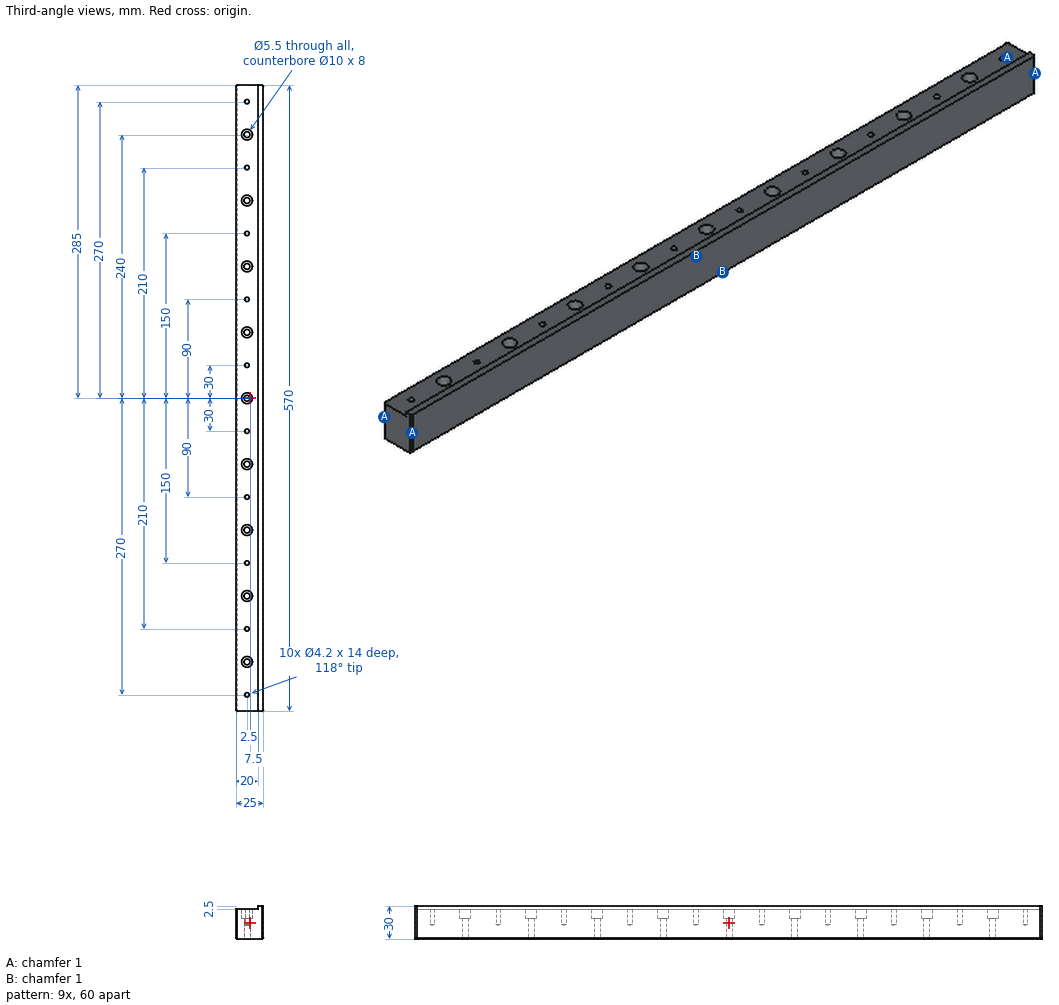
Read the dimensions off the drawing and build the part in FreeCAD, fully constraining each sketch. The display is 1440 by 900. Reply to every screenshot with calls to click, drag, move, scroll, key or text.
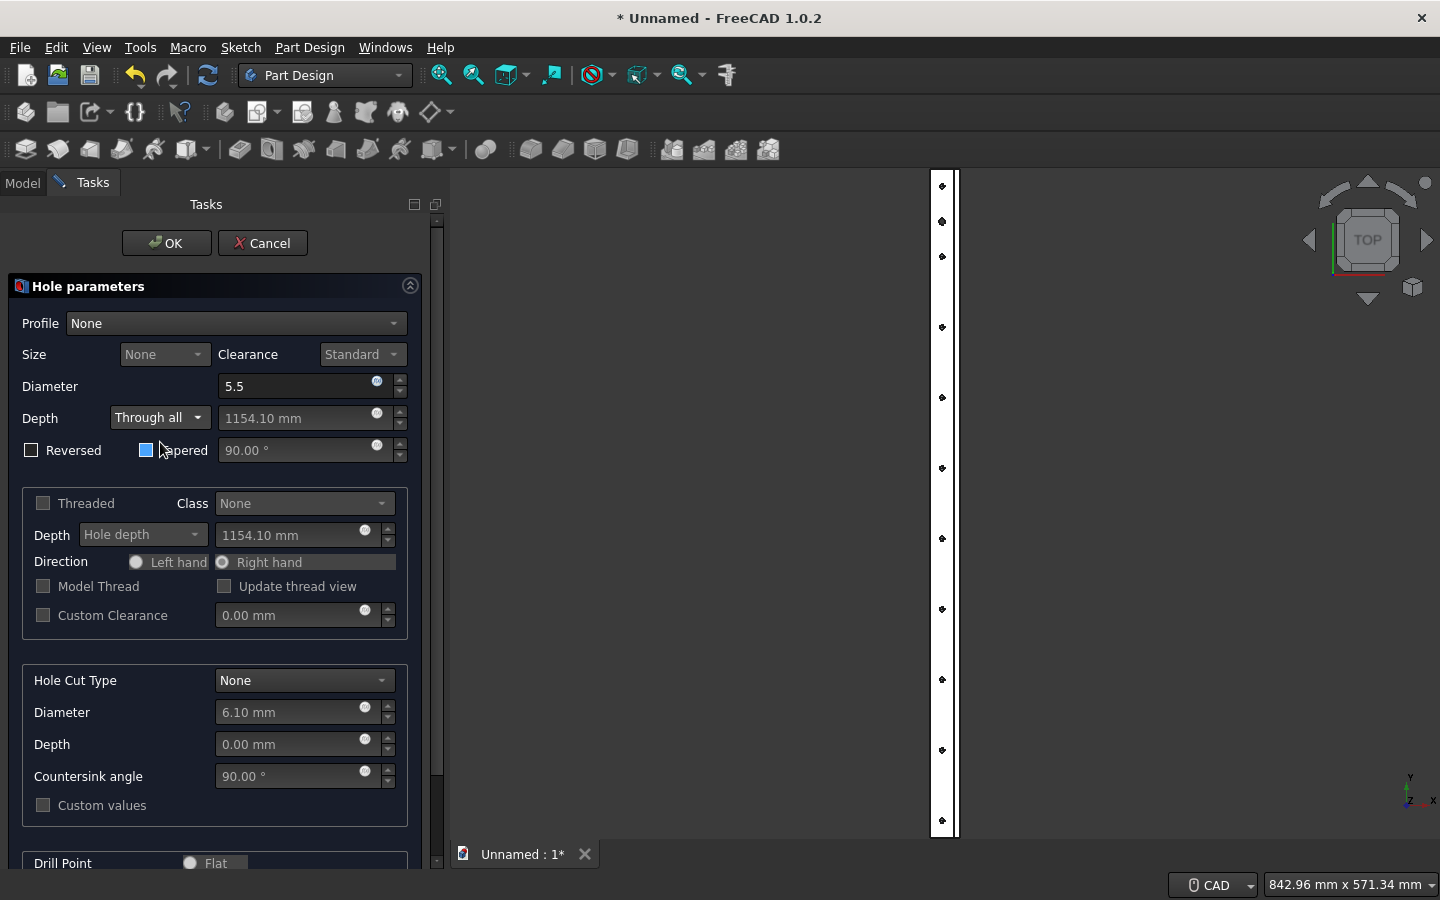
click(306, 680)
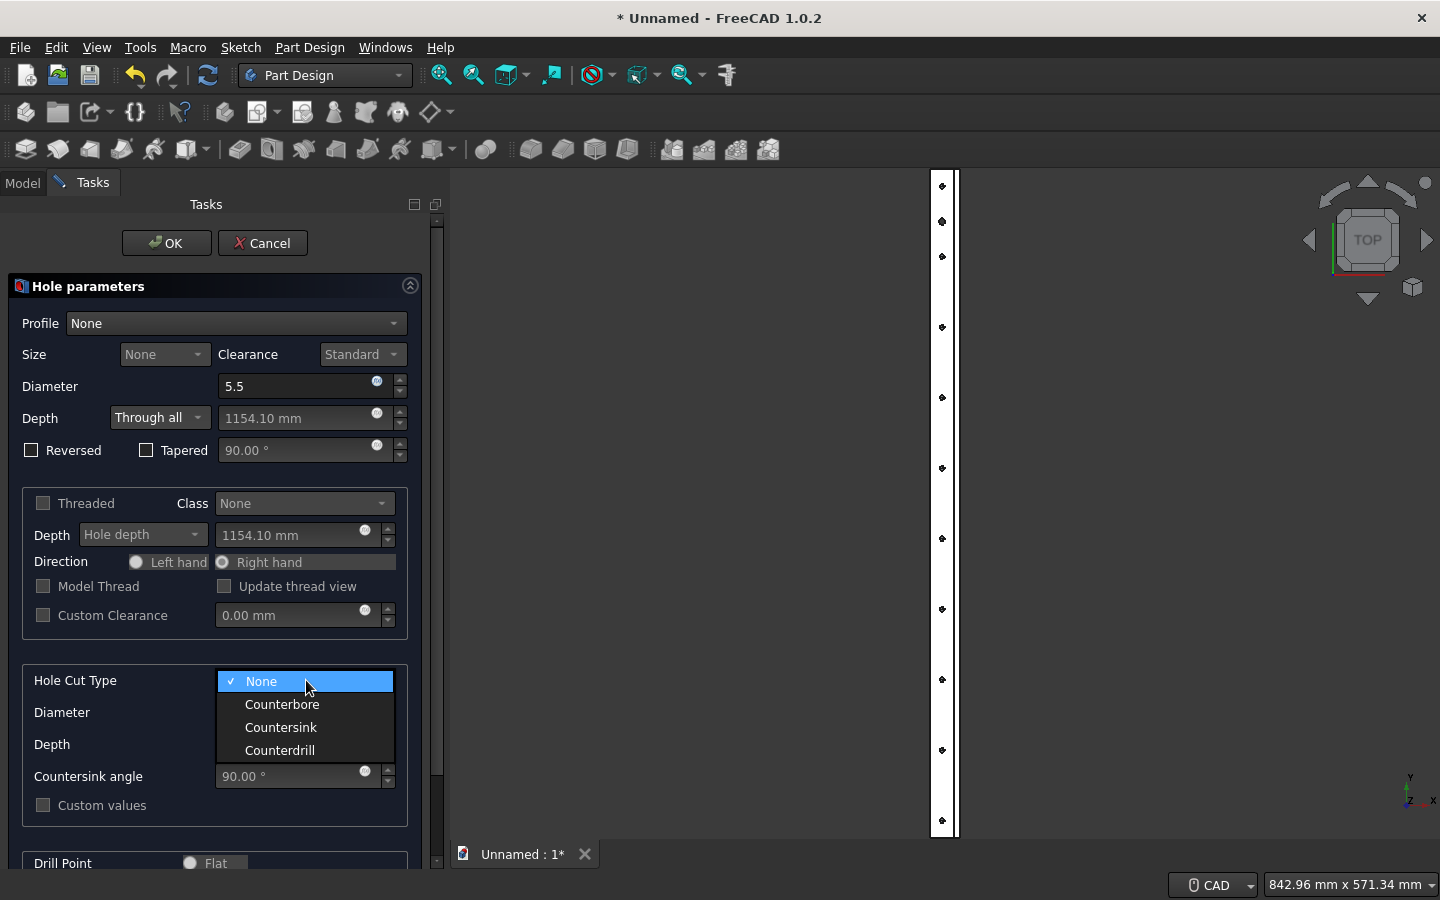
click(304, 704)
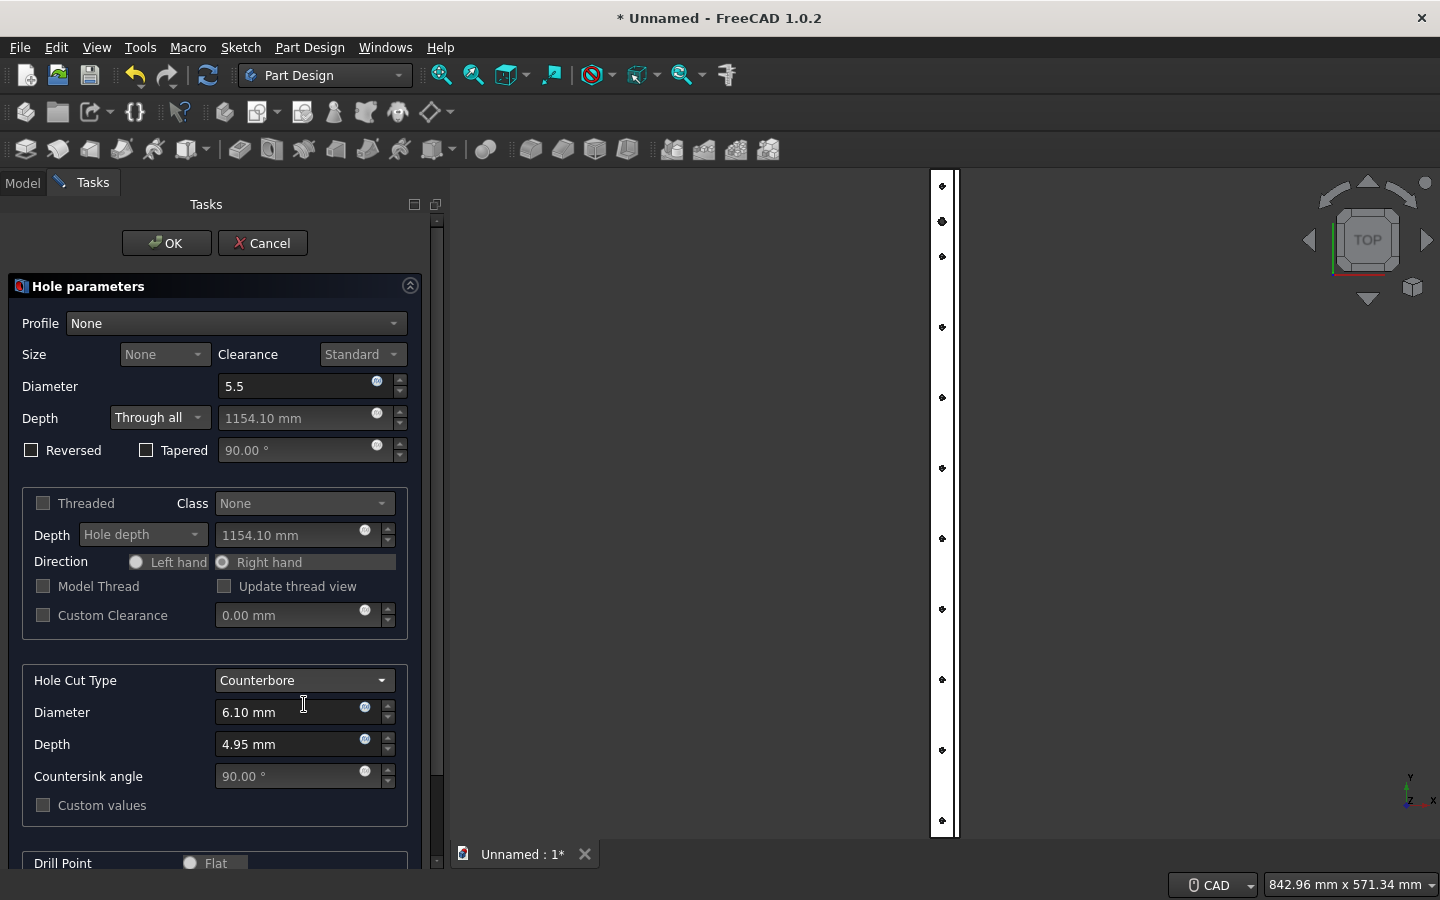
triple_click(298, 712)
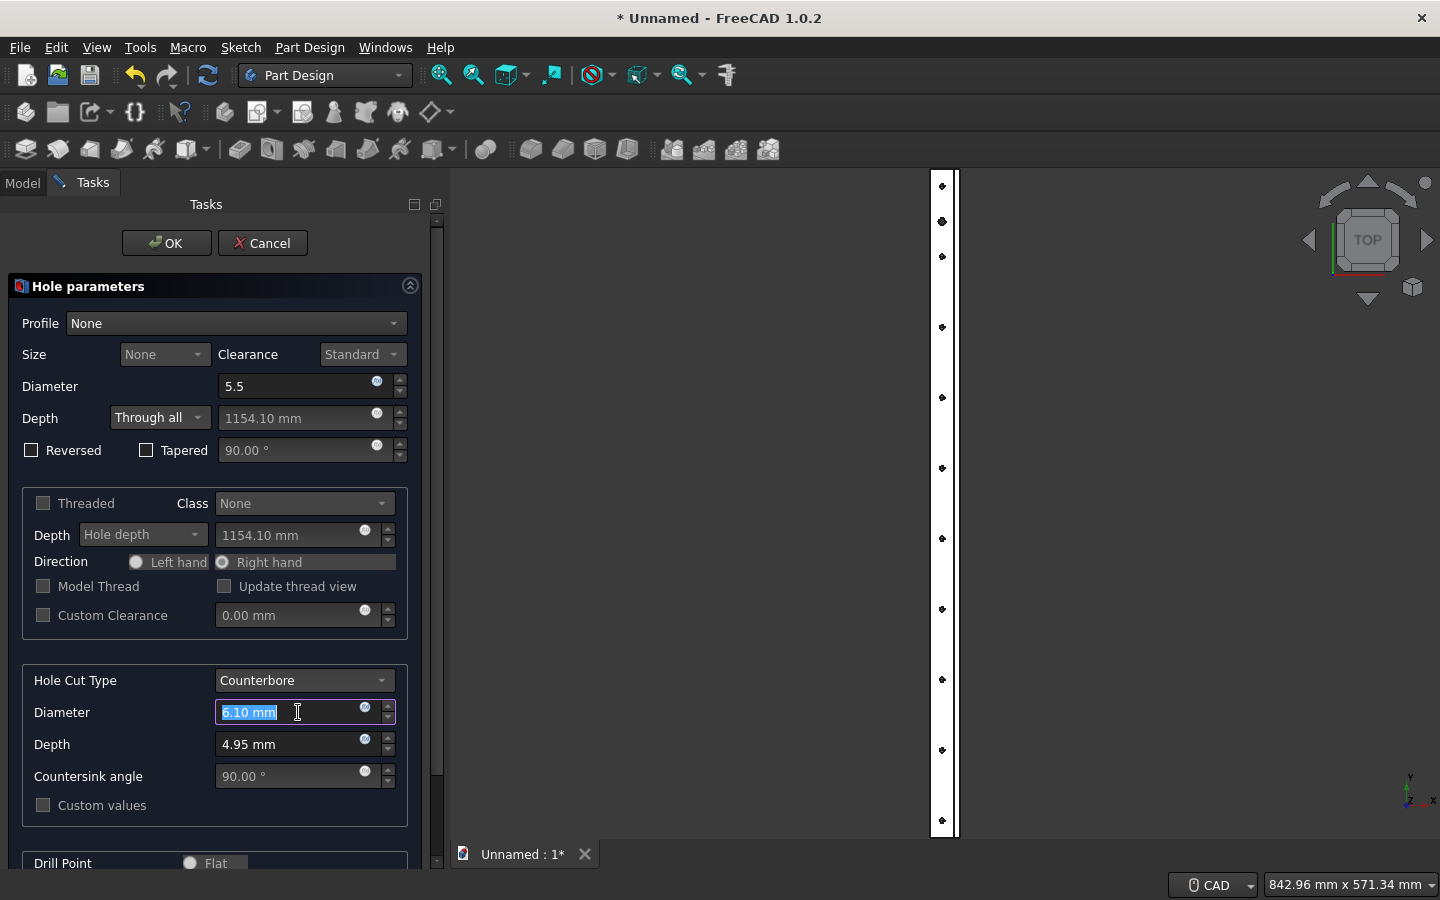
text(10)
key(Tab)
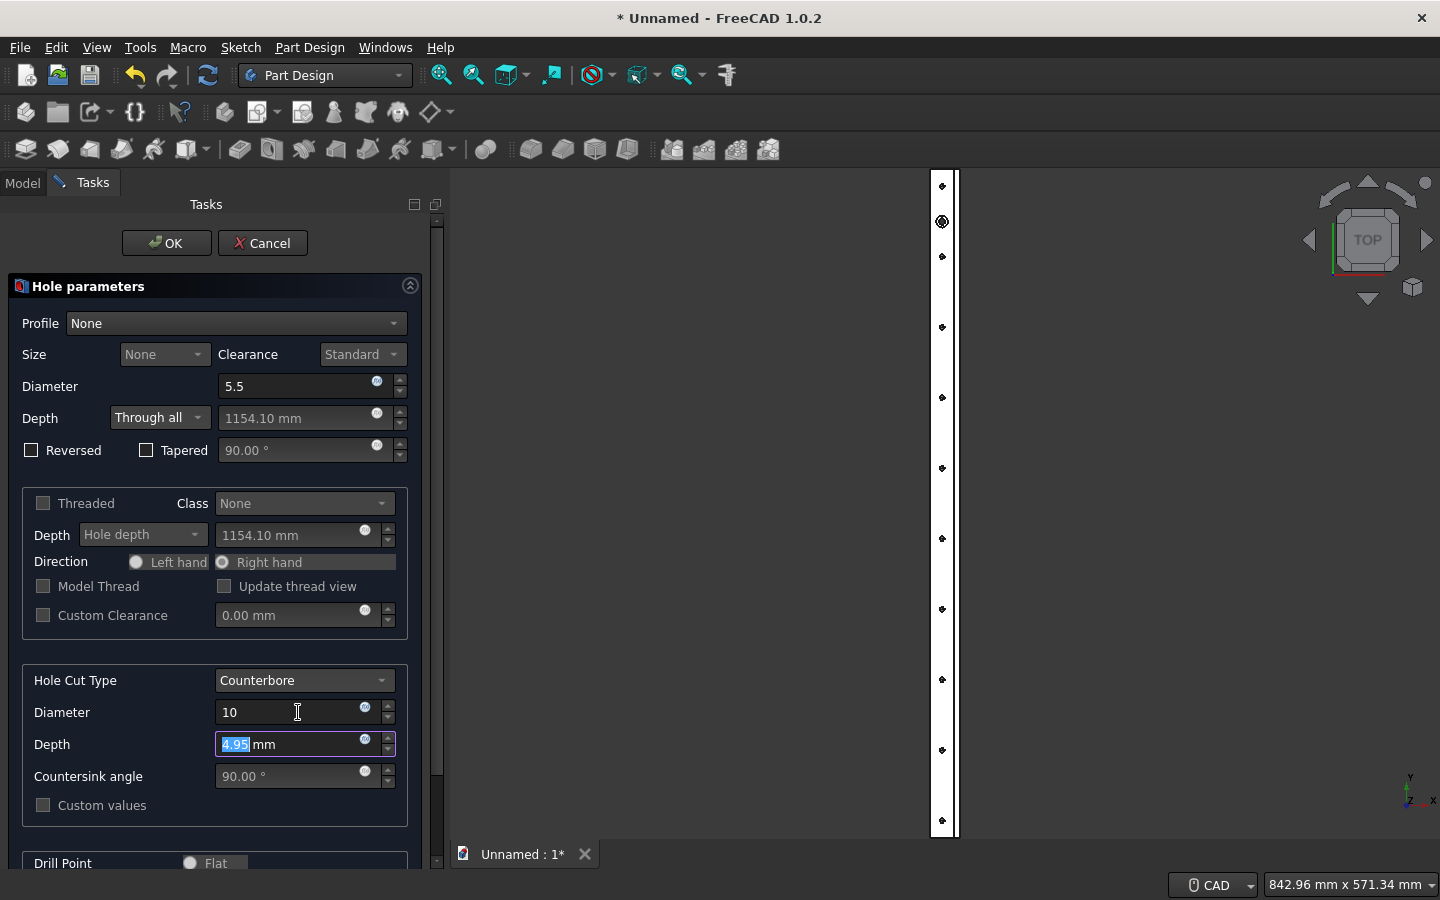
text(8)
key(Tab)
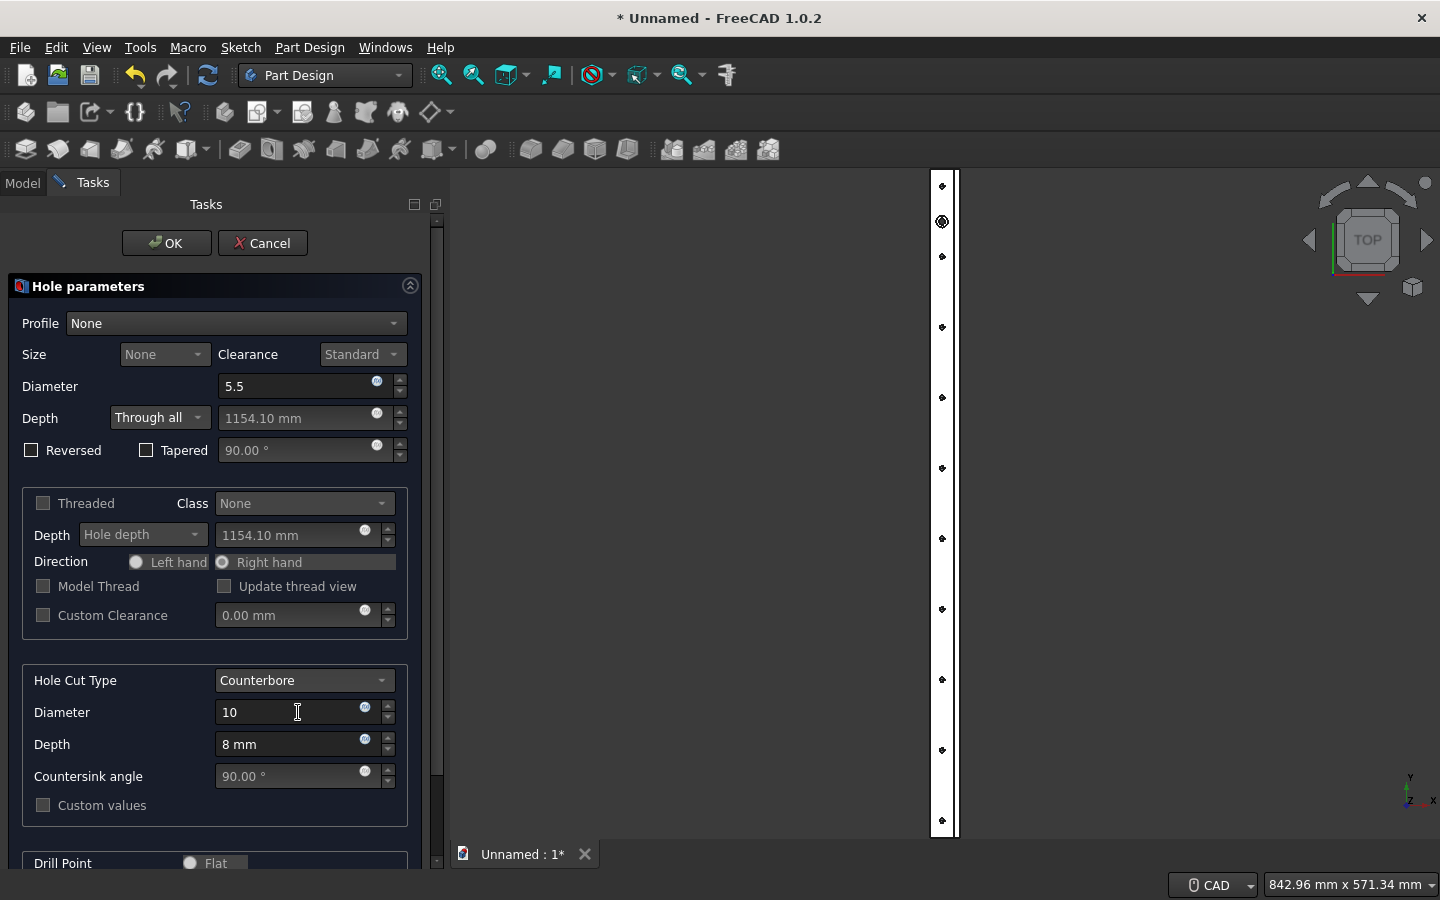
click(167, 243)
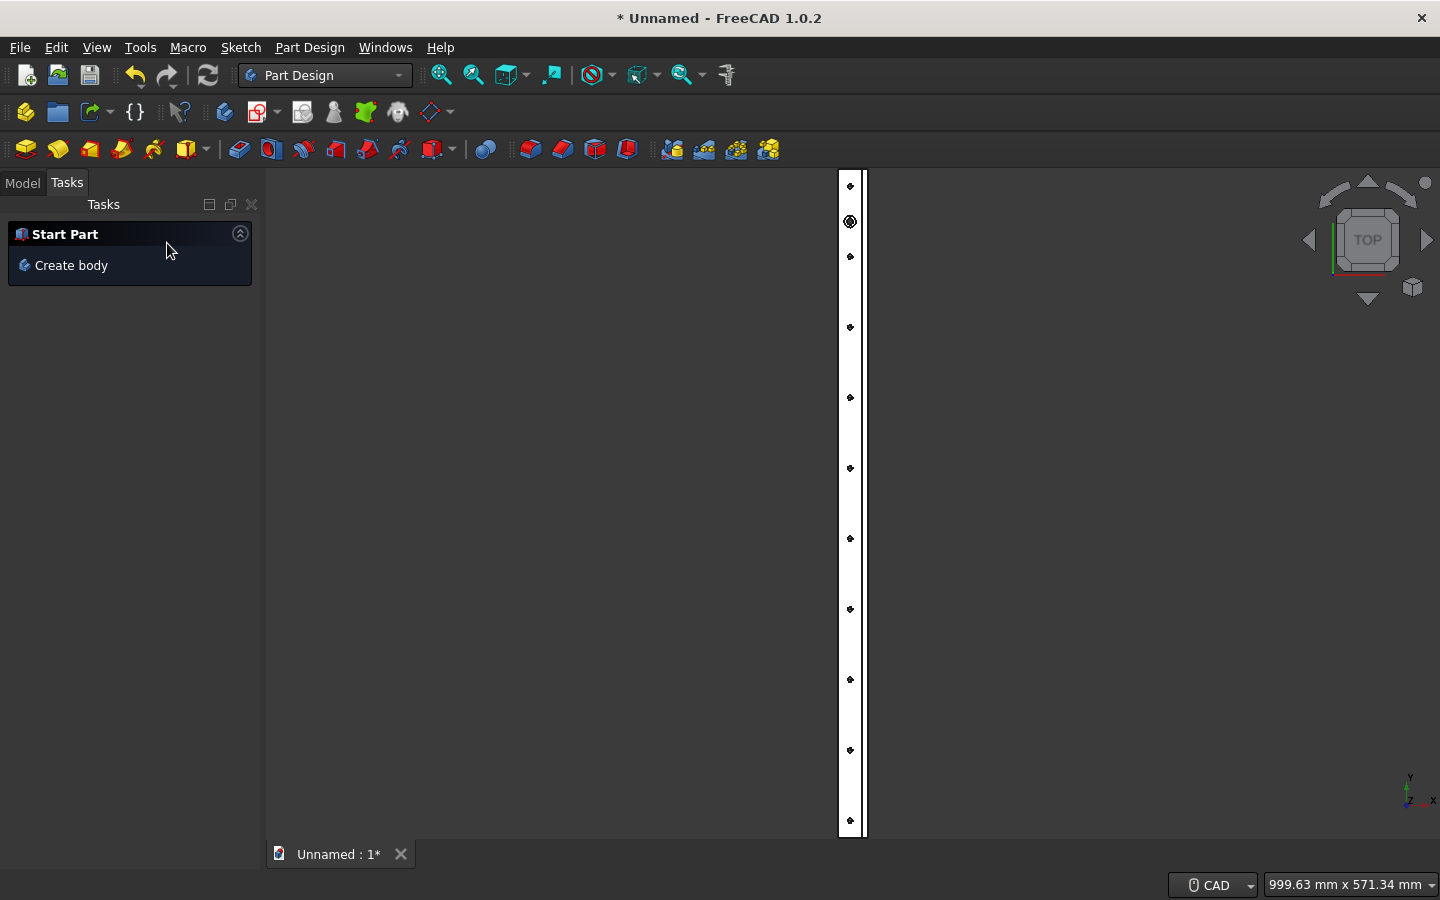
click(23, 182)